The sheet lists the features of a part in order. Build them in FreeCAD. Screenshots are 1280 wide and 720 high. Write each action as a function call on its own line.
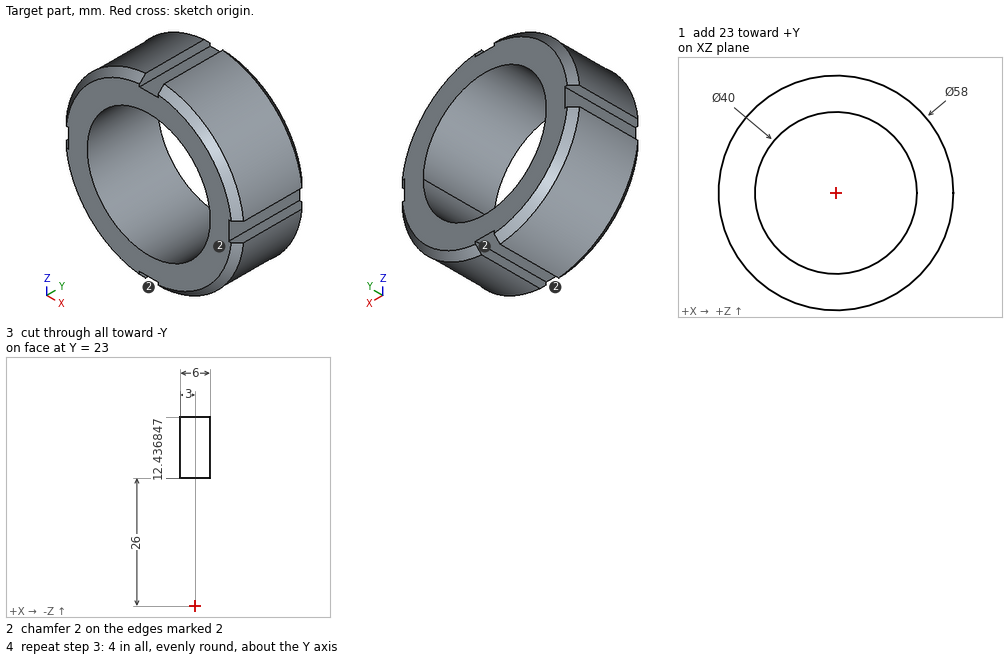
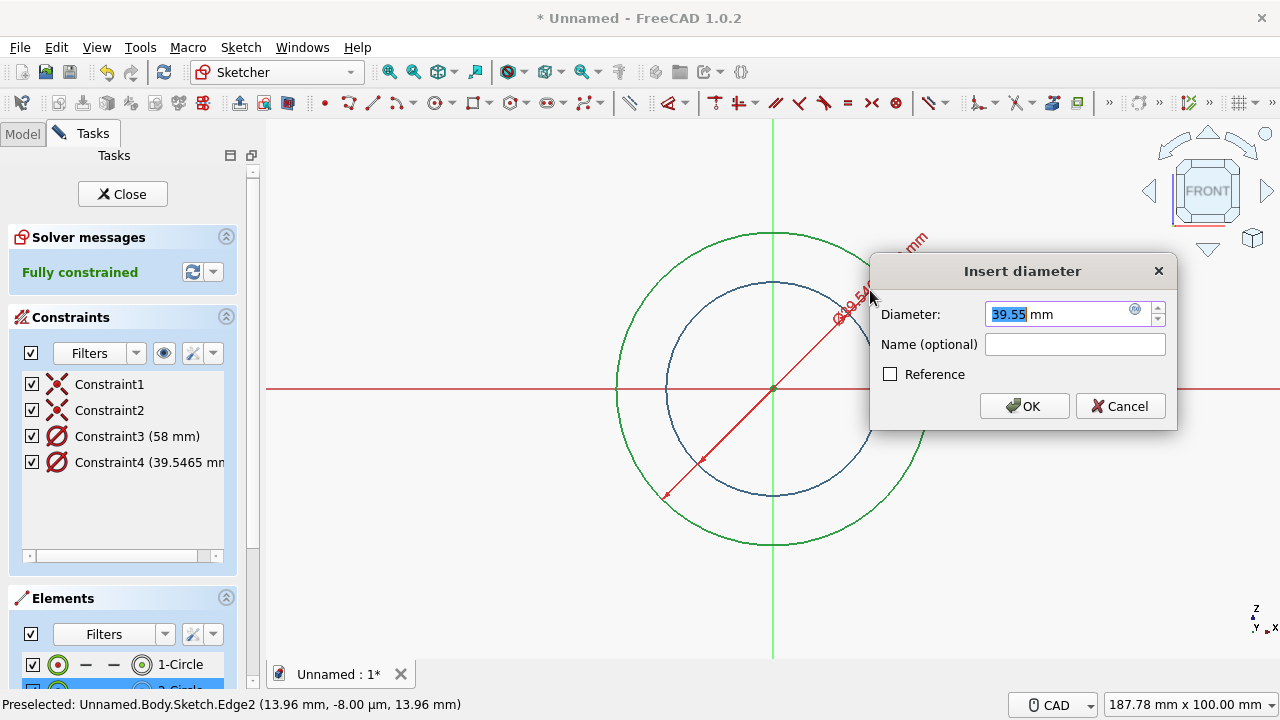
text(40)
key(Return)
key(Escape)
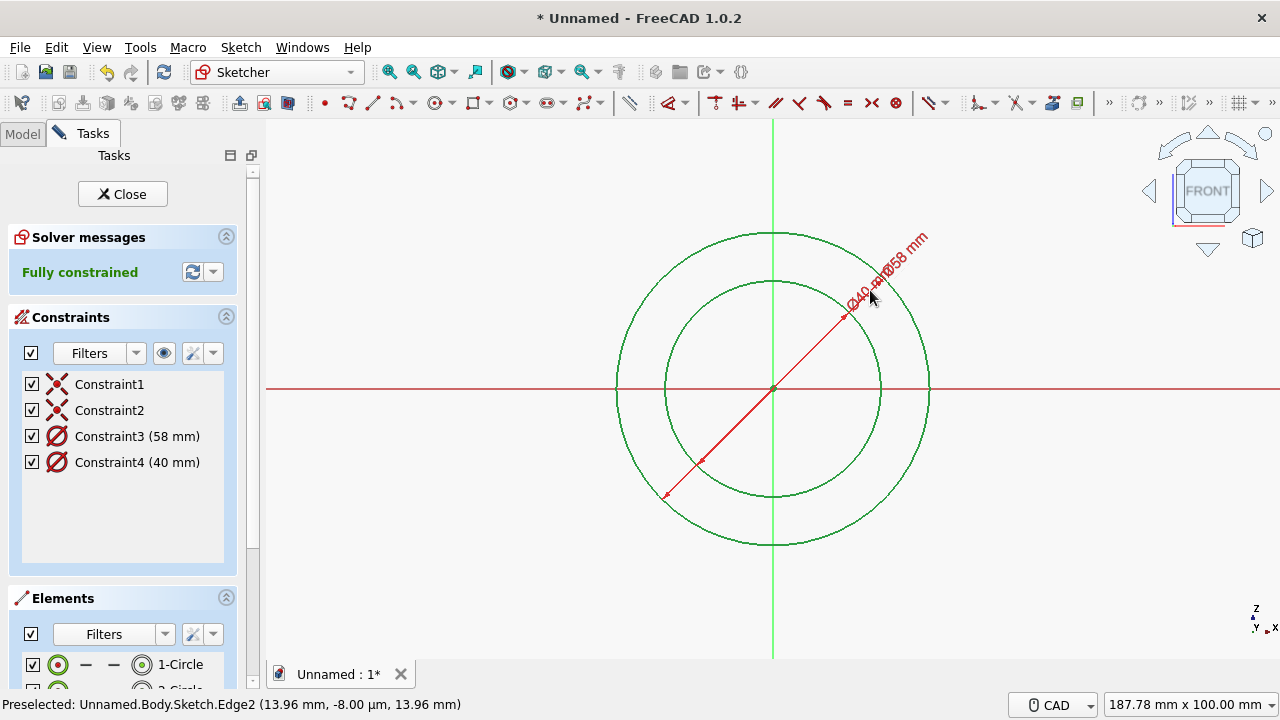
click(123, 194)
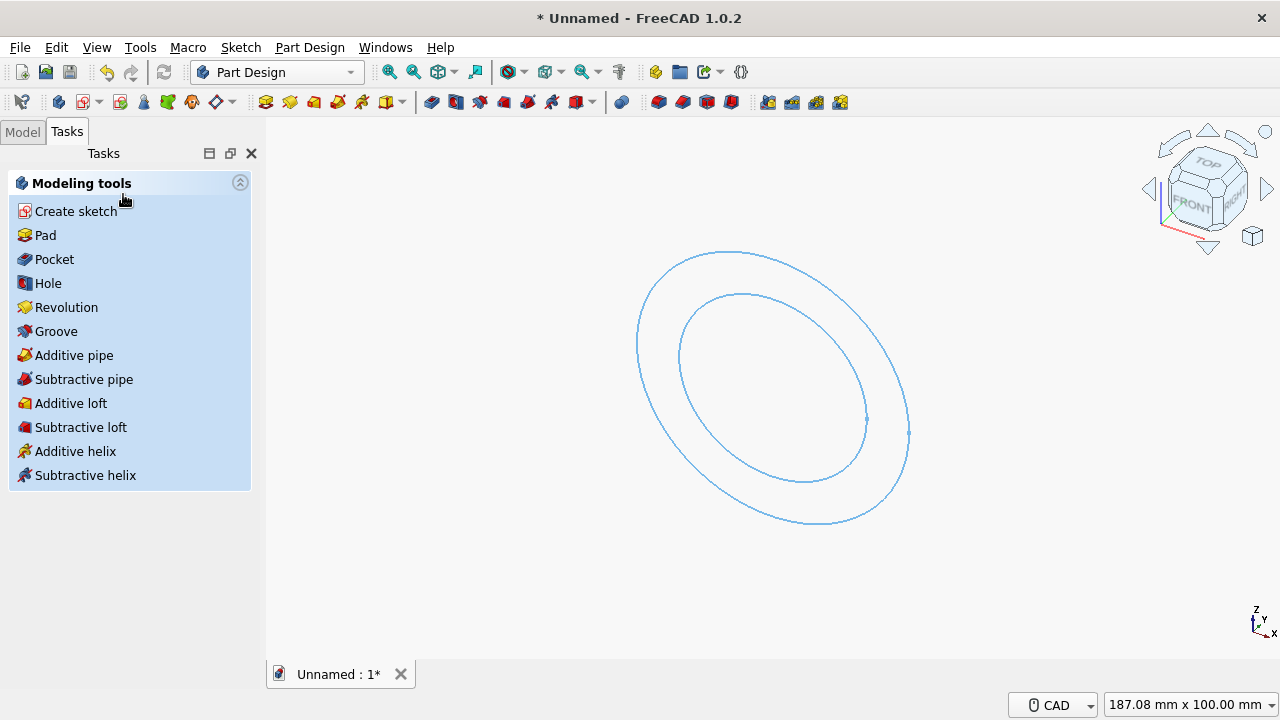
click(266, 102)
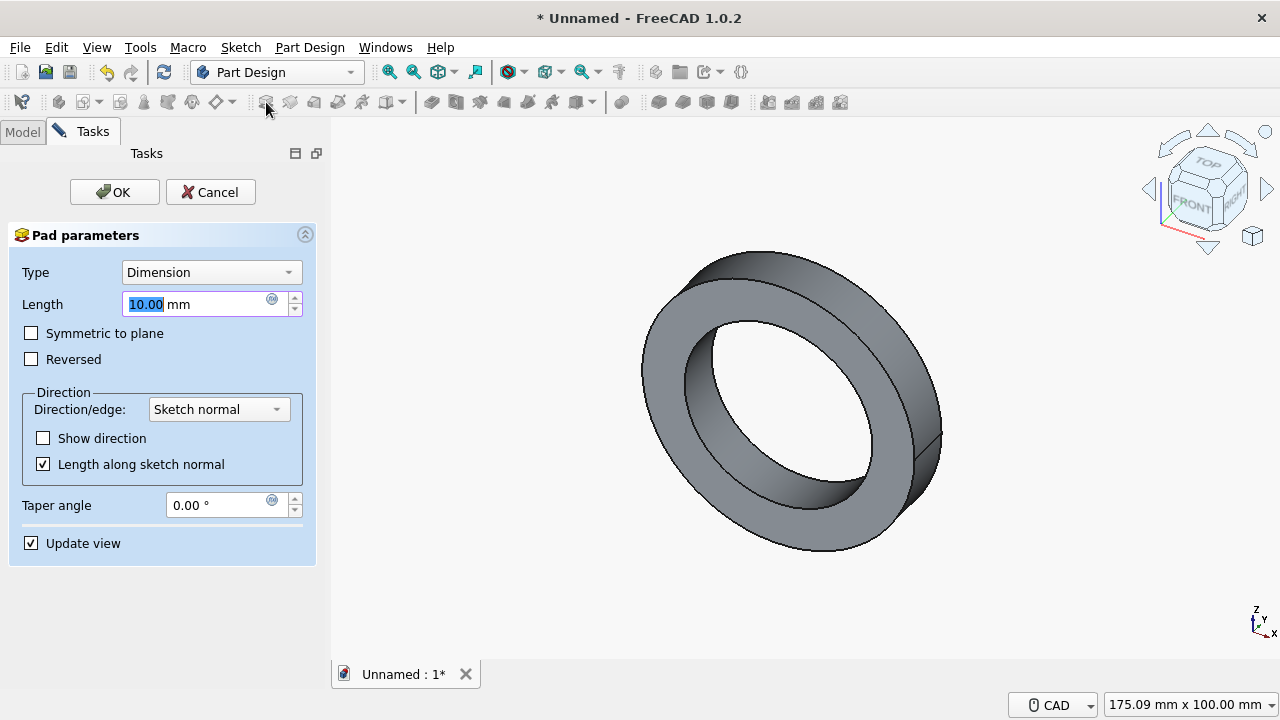
text(23)
key(Tab)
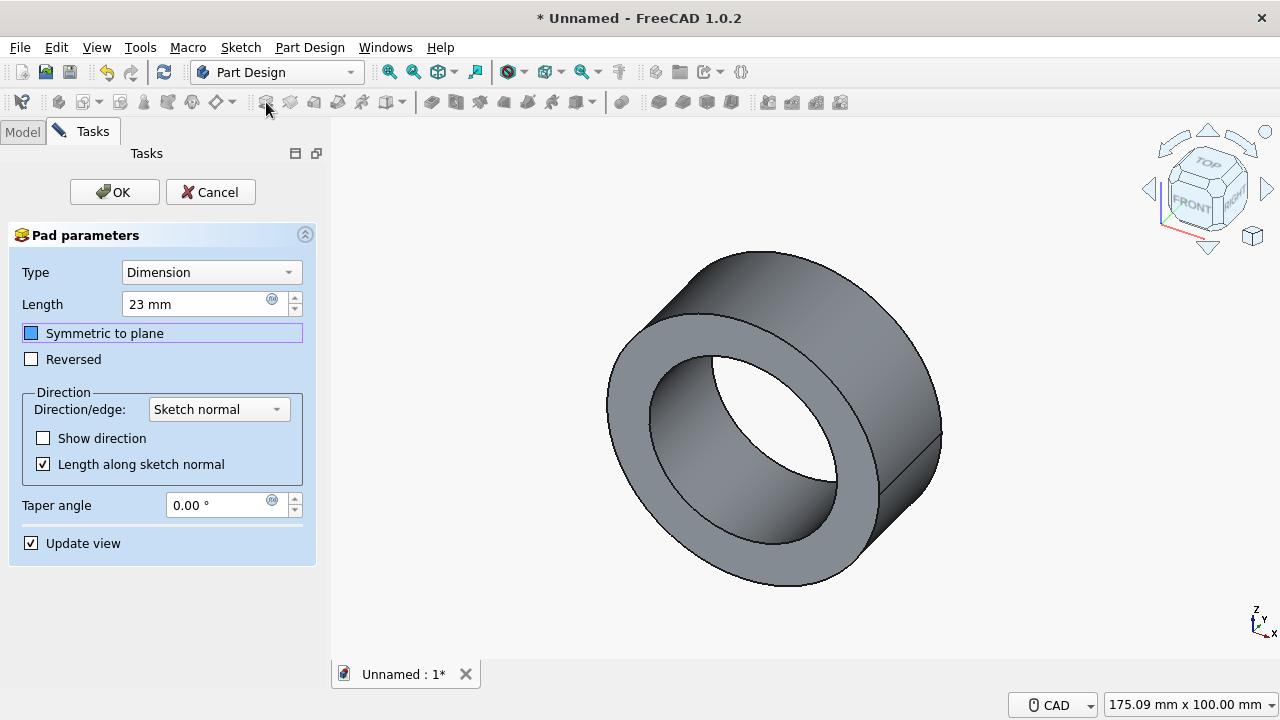
click(30, 359)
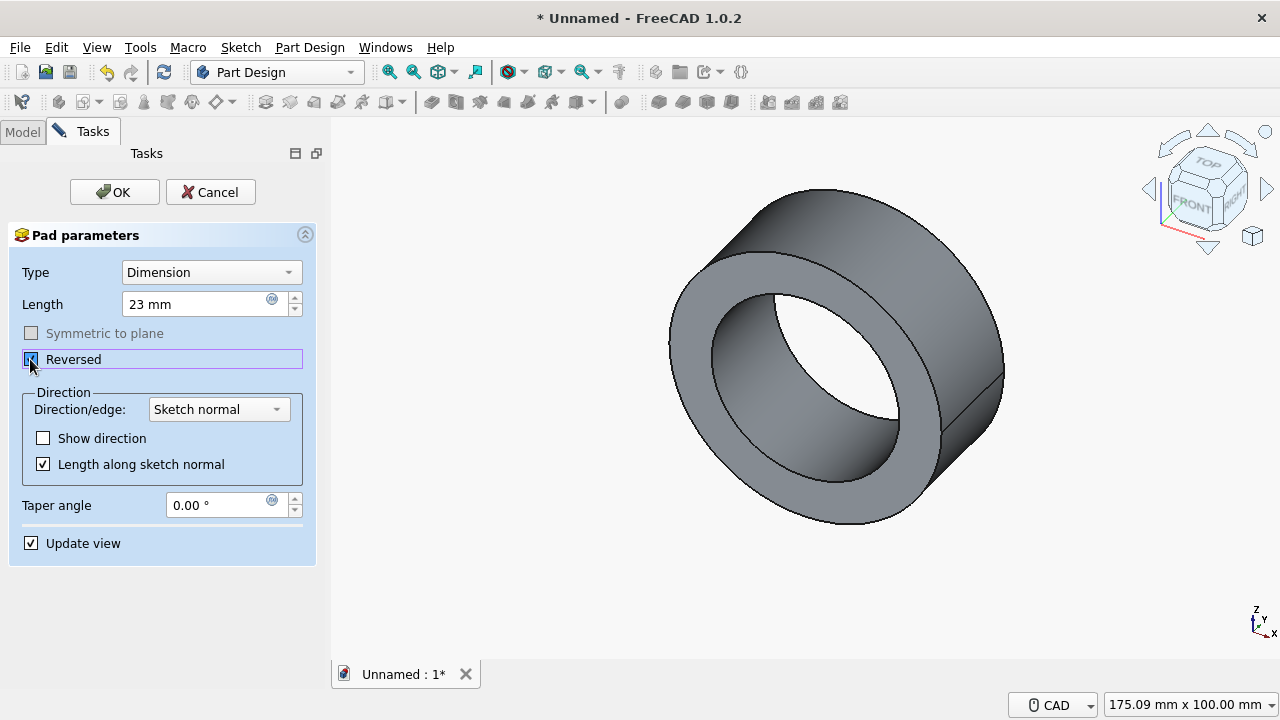
click(115, 192)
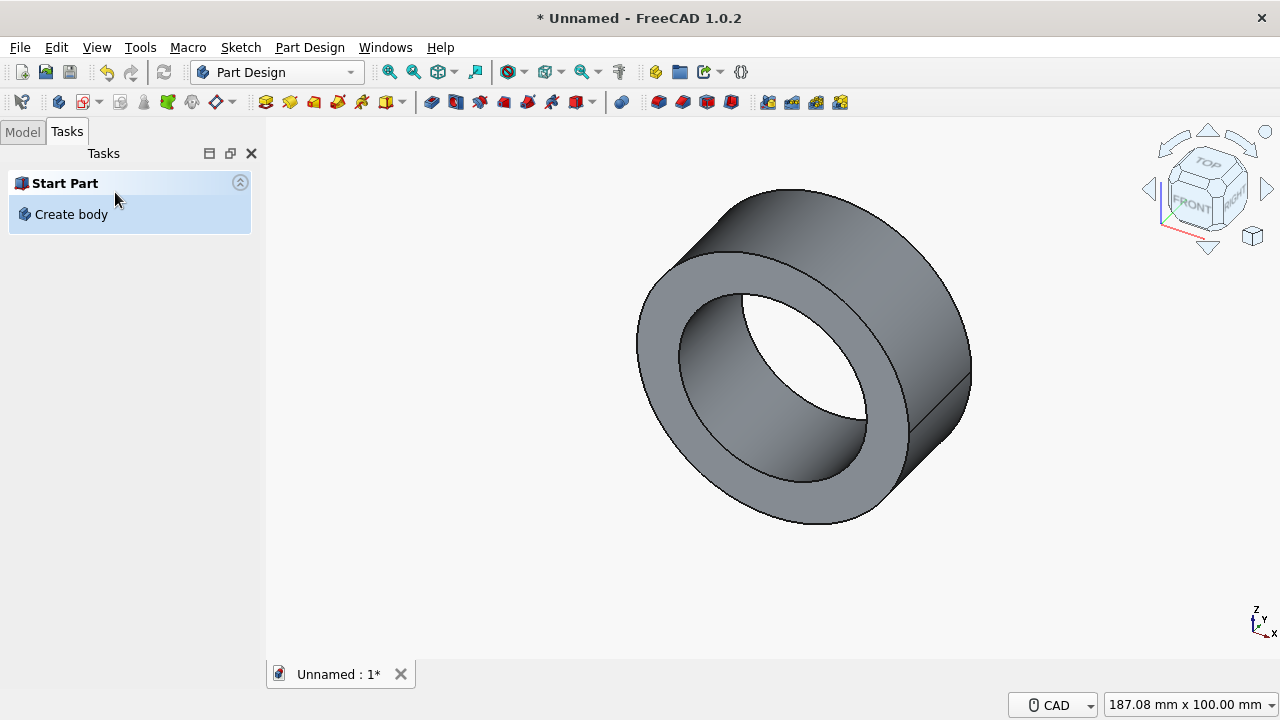
click(731, 251)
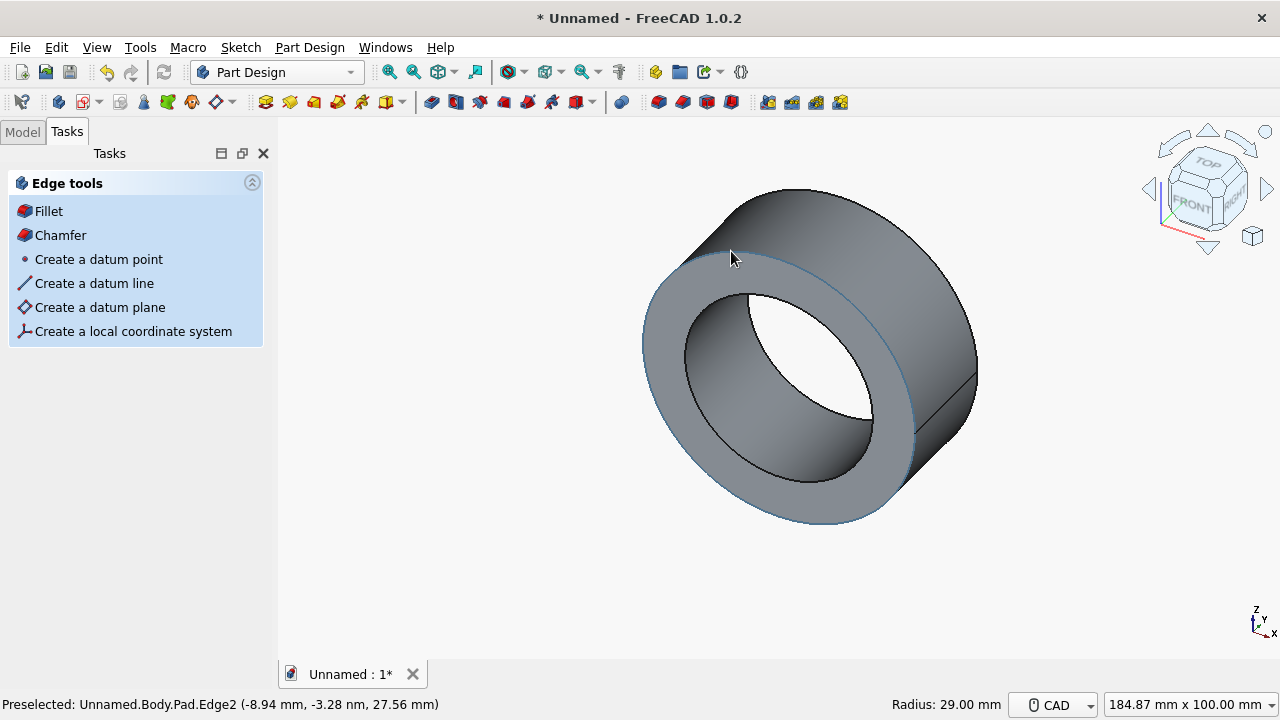
key(0)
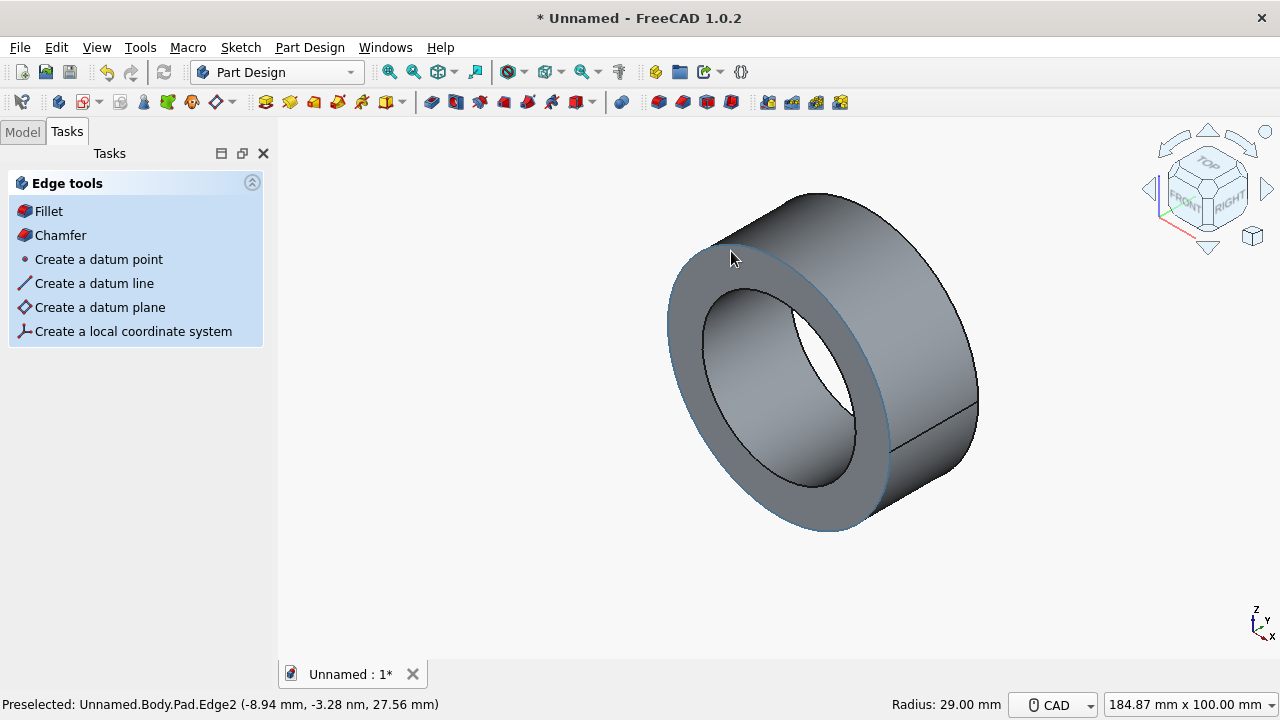
key(2)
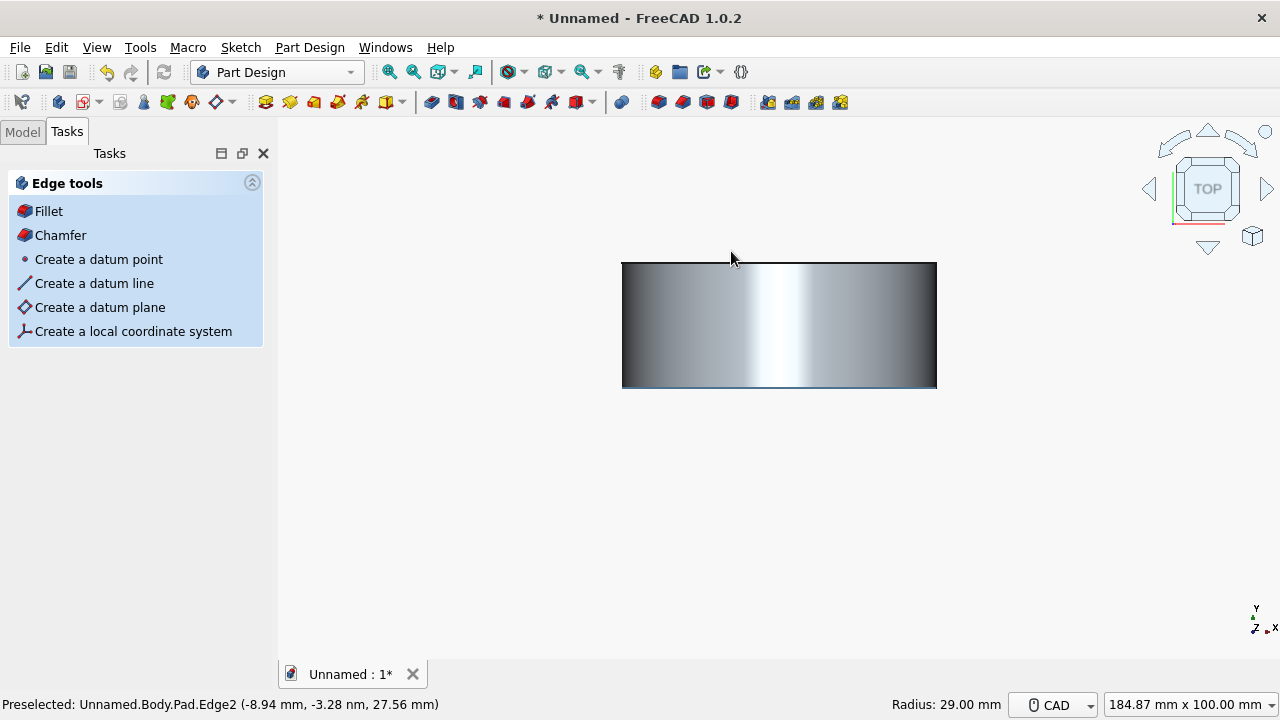
click(390, 72)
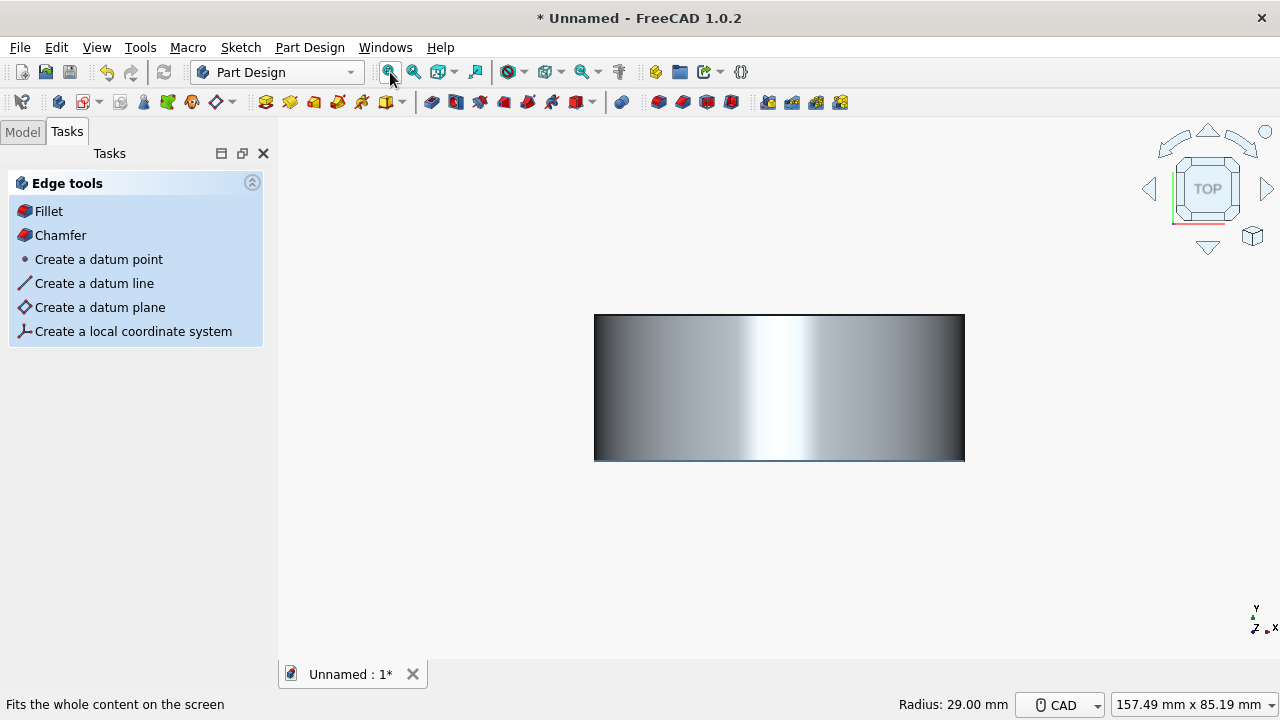
click(630, 314, ctrl)